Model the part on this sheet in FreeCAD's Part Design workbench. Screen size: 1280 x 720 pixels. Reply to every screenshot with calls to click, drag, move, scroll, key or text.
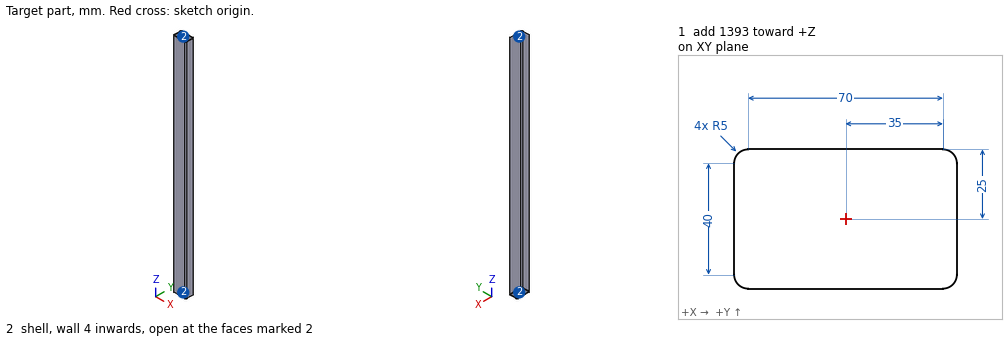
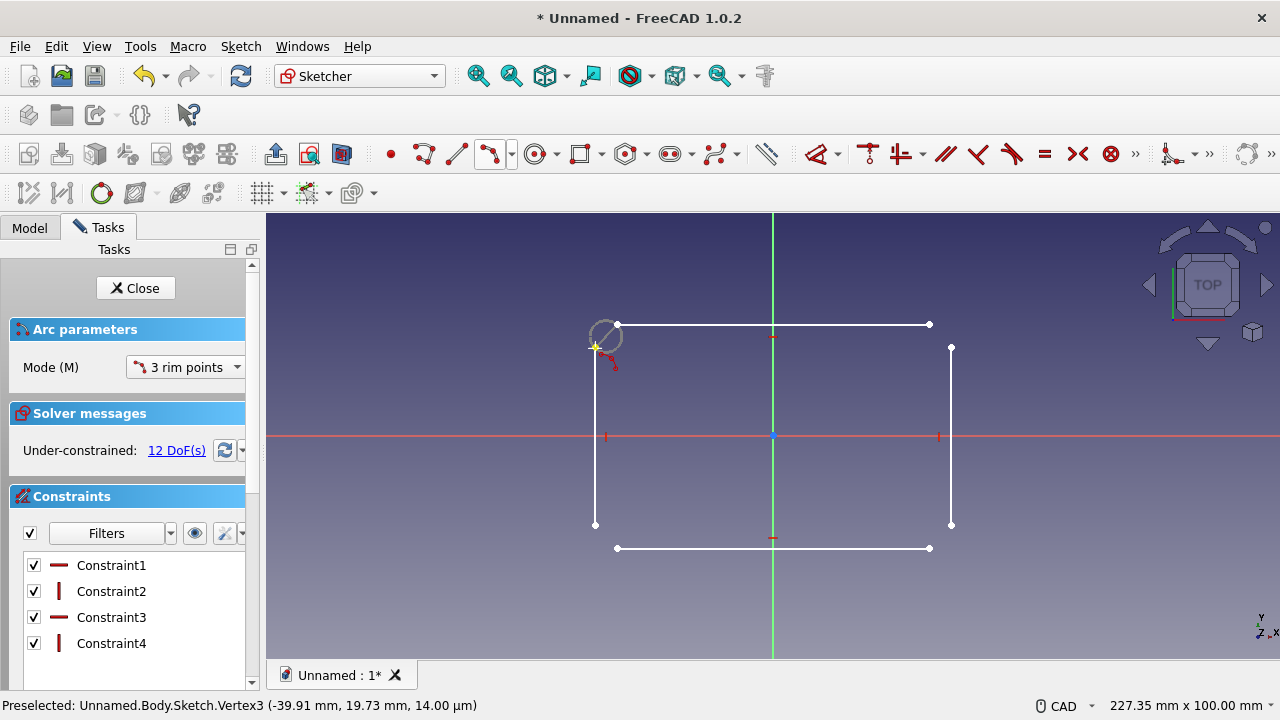
scroll(601, 331, up, 5)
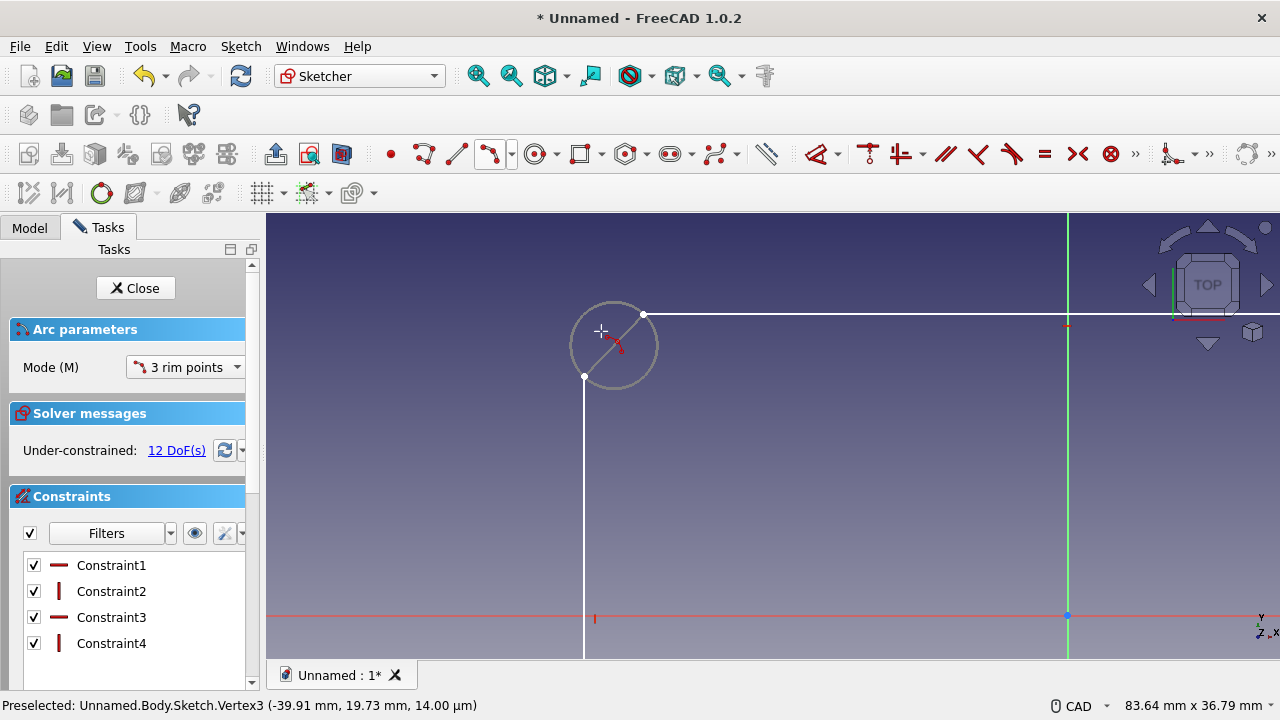
click(601, 331)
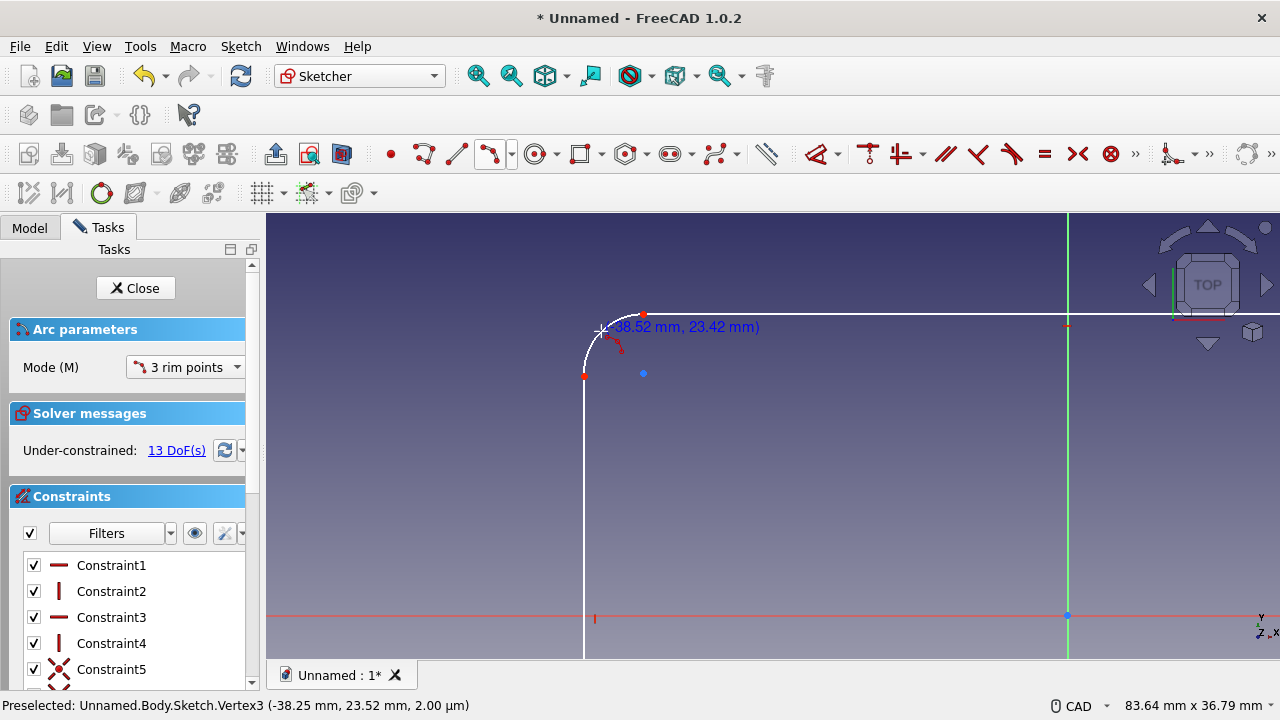
scroll(408, 289, down, 4)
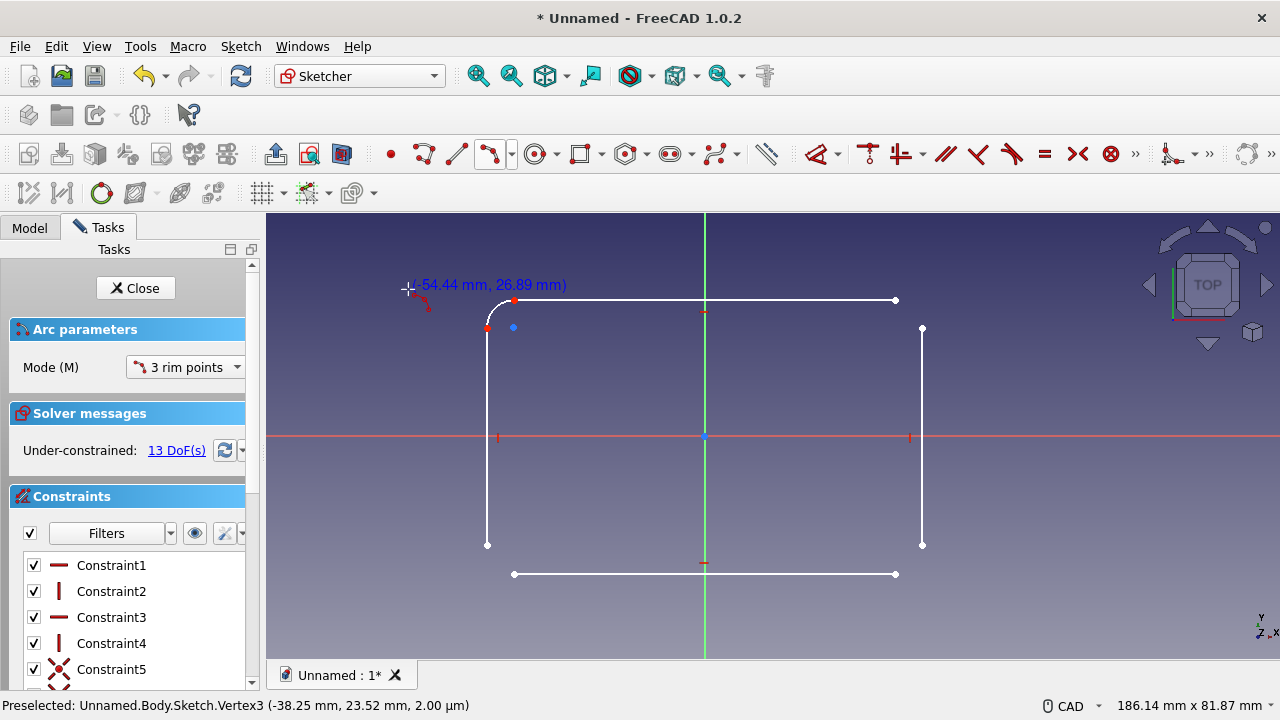
click(487, 546)
click(514, 574)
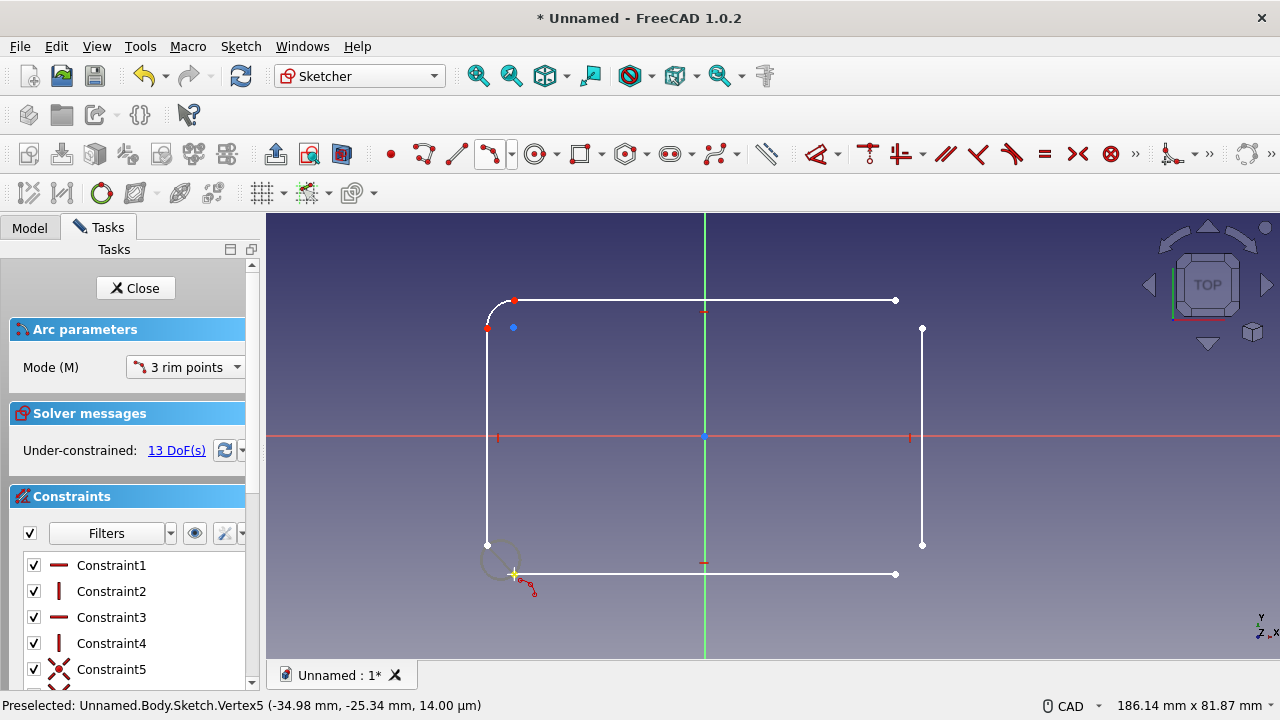
scroll(495, 564, up, 4)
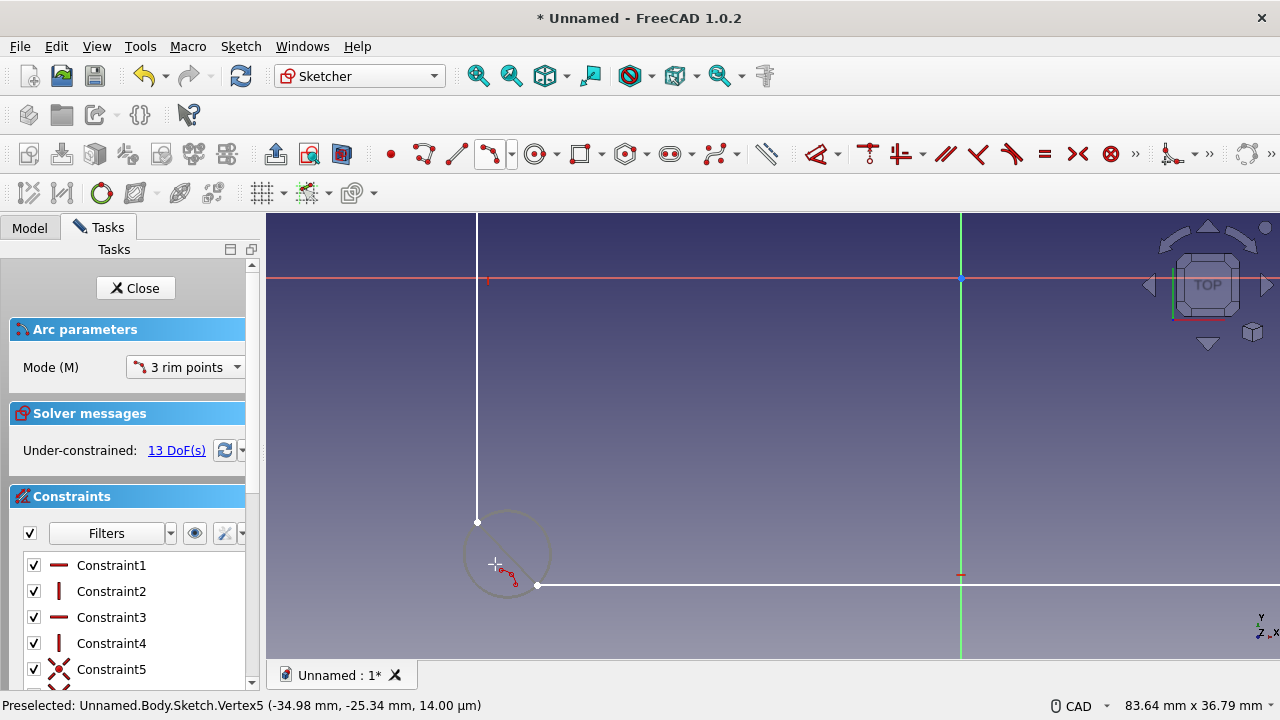
click(494, 564)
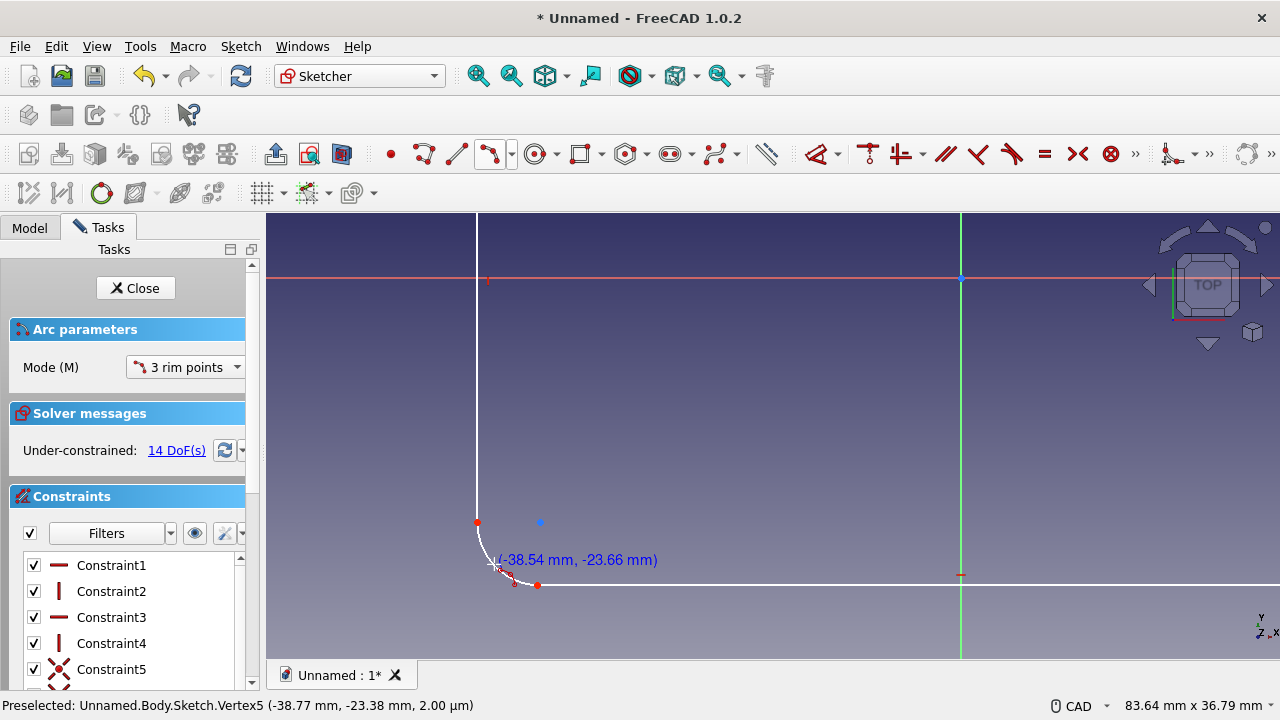
scroll(495, 565, down, 4)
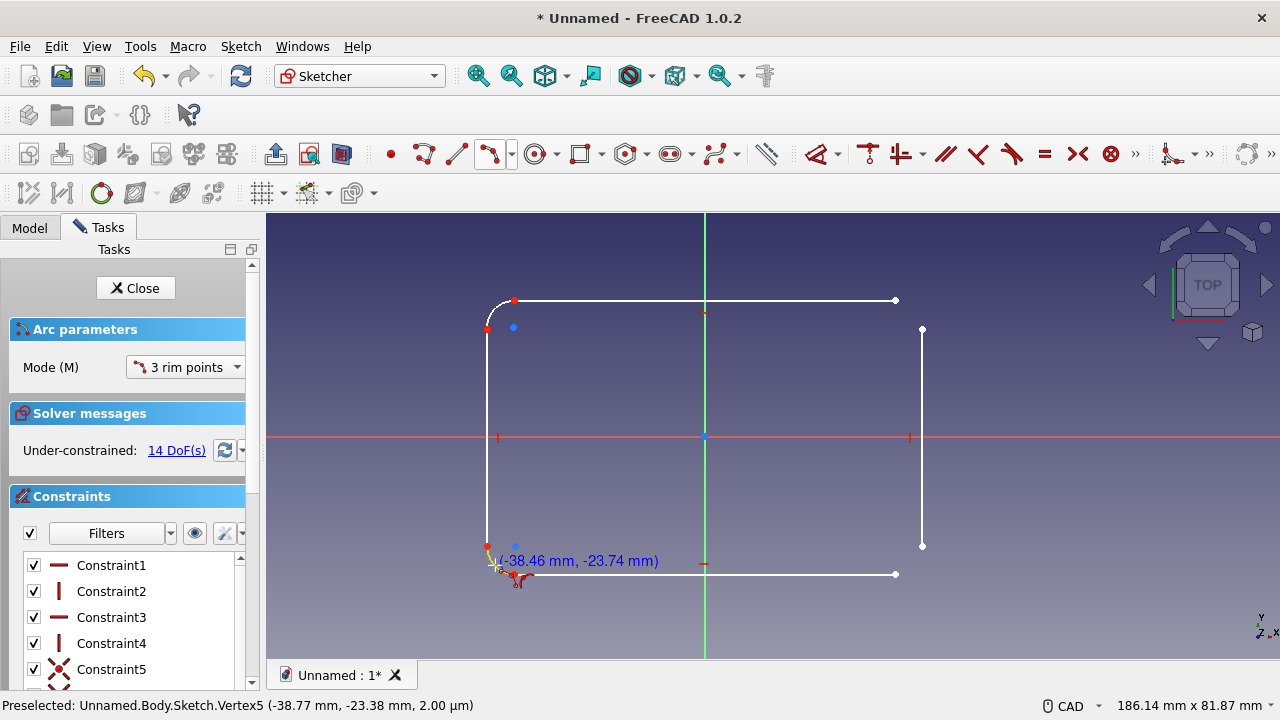
click(895, 575)
click(922, 546)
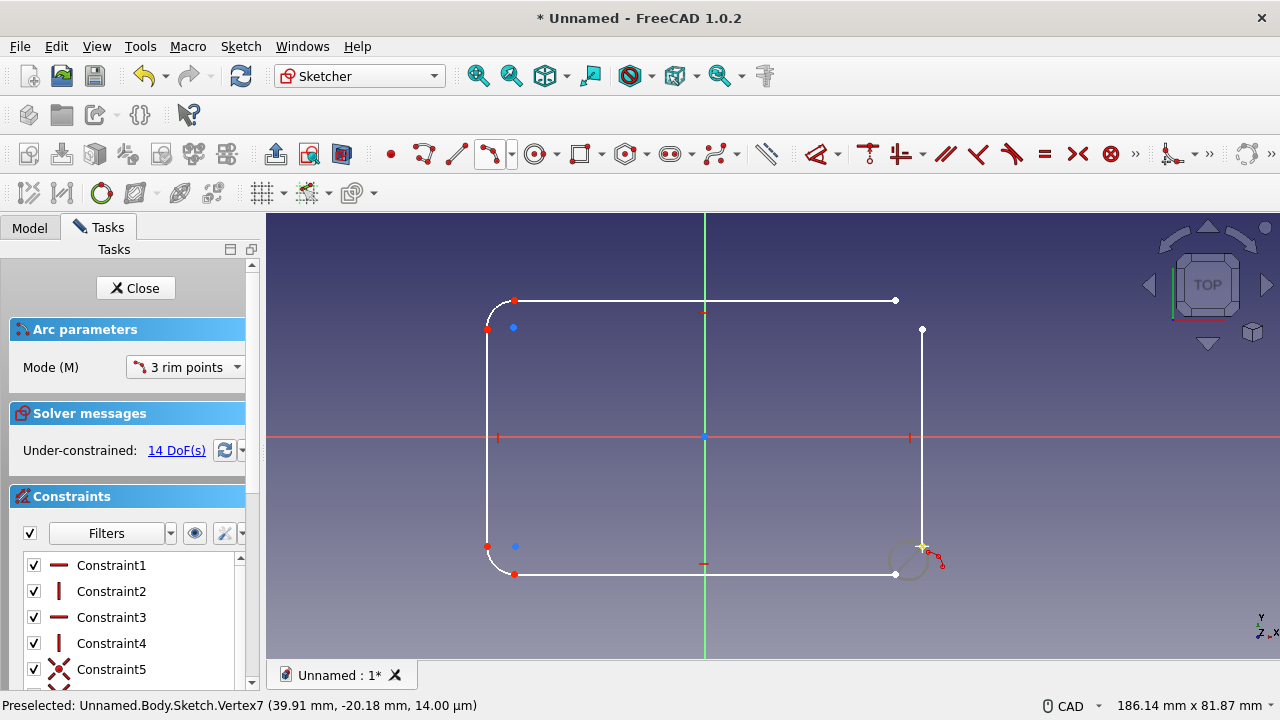
scroll(915, 565, up, 4)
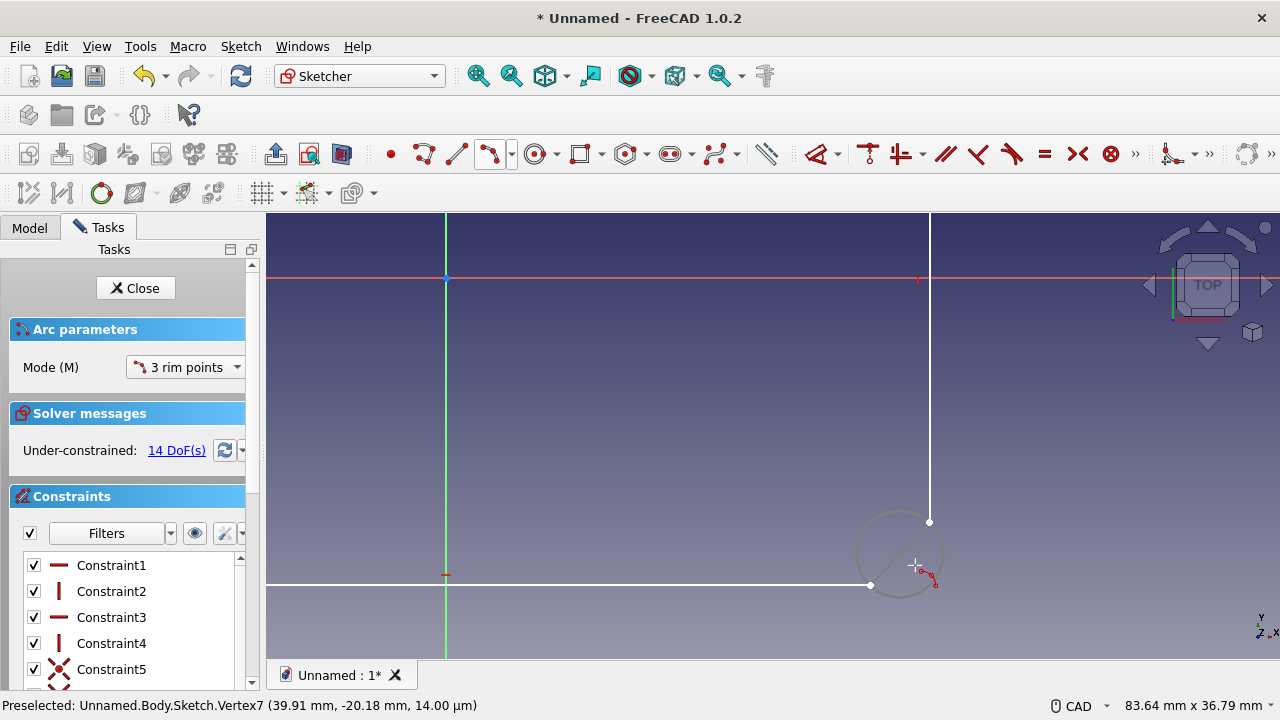
click(913, 564)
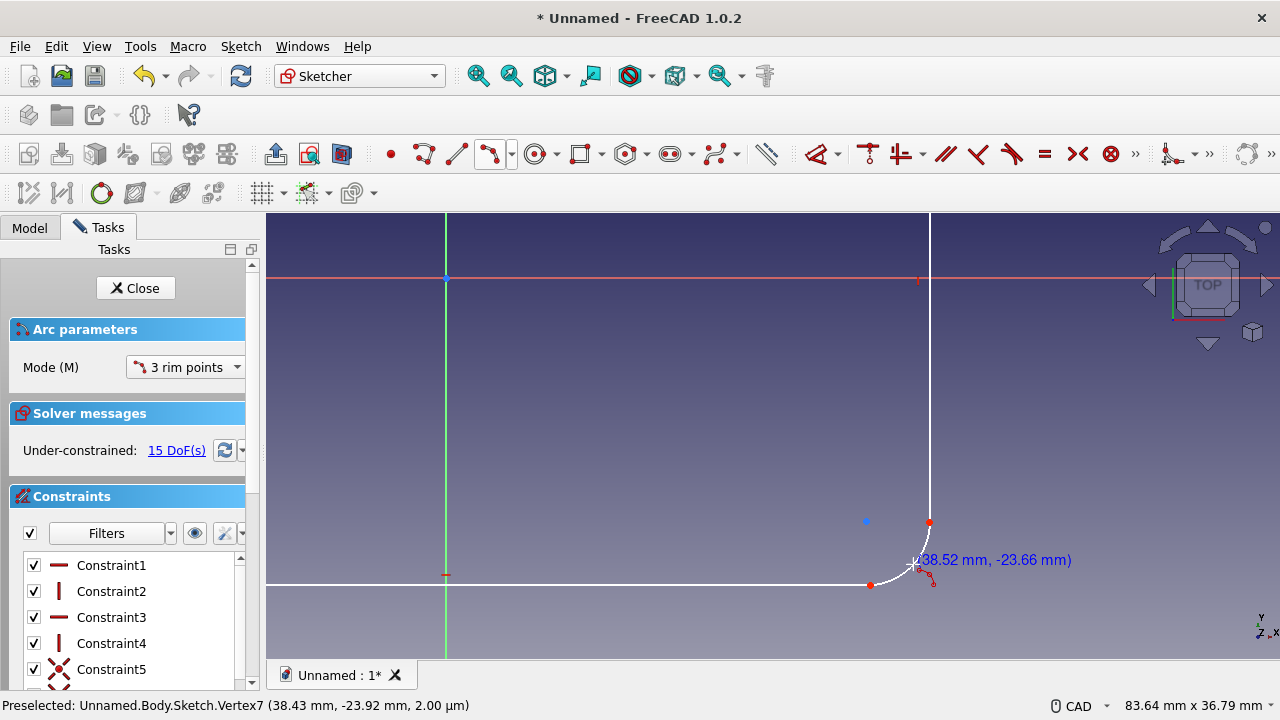
scroll(915, 565, down, 4)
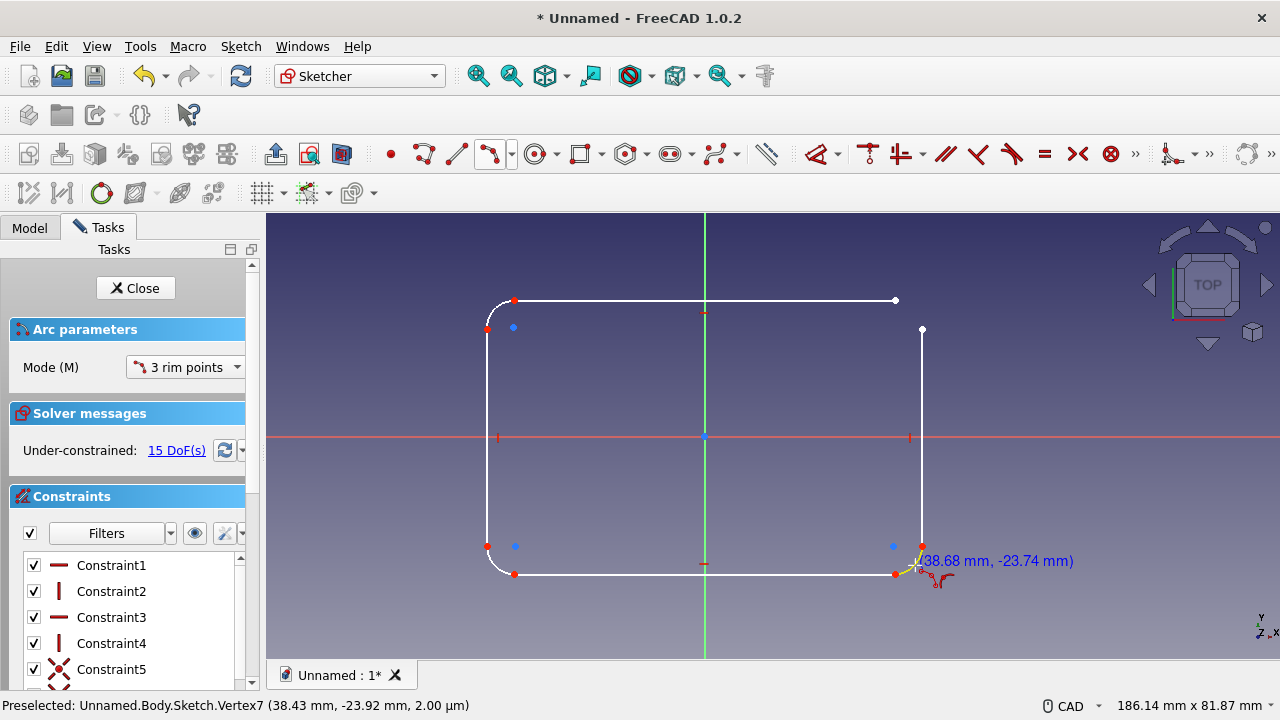
click(922, 329)
click(895, 301)